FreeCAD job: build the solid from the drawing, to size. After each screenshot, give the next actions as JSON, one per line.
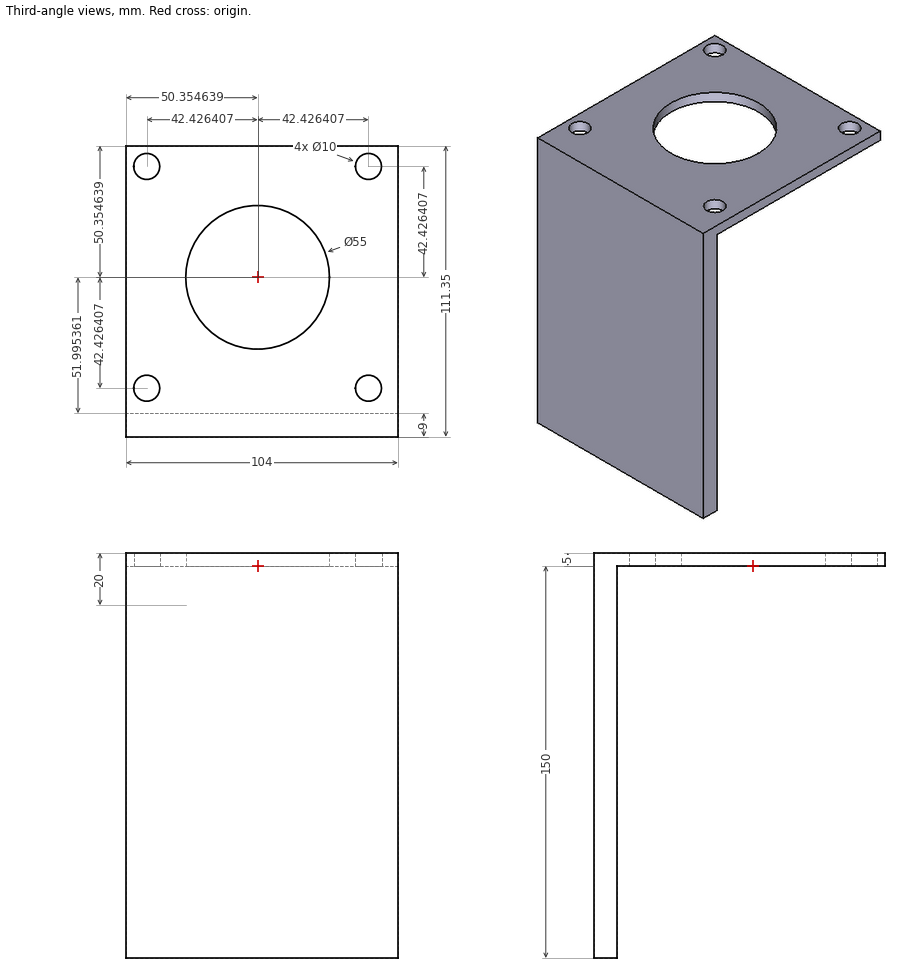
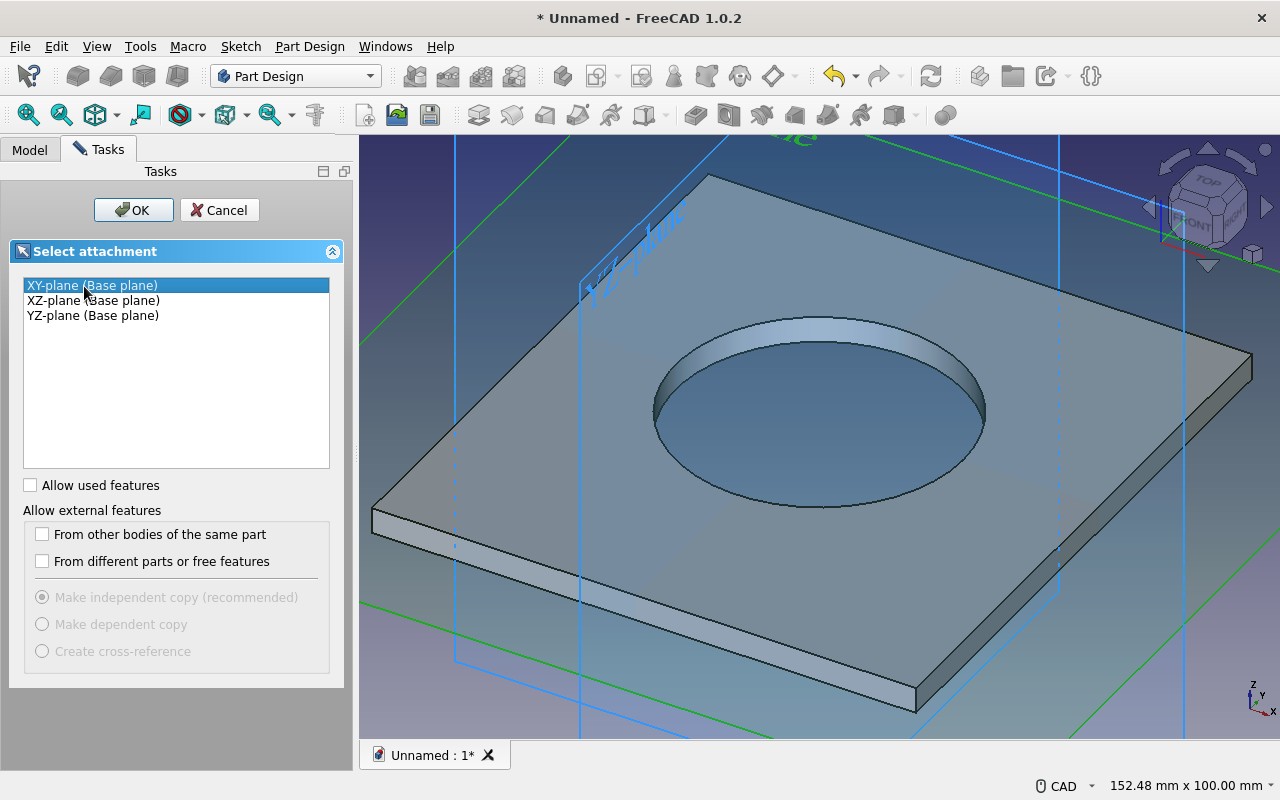
{"action": "left_click", "coordinate": [134, 210]}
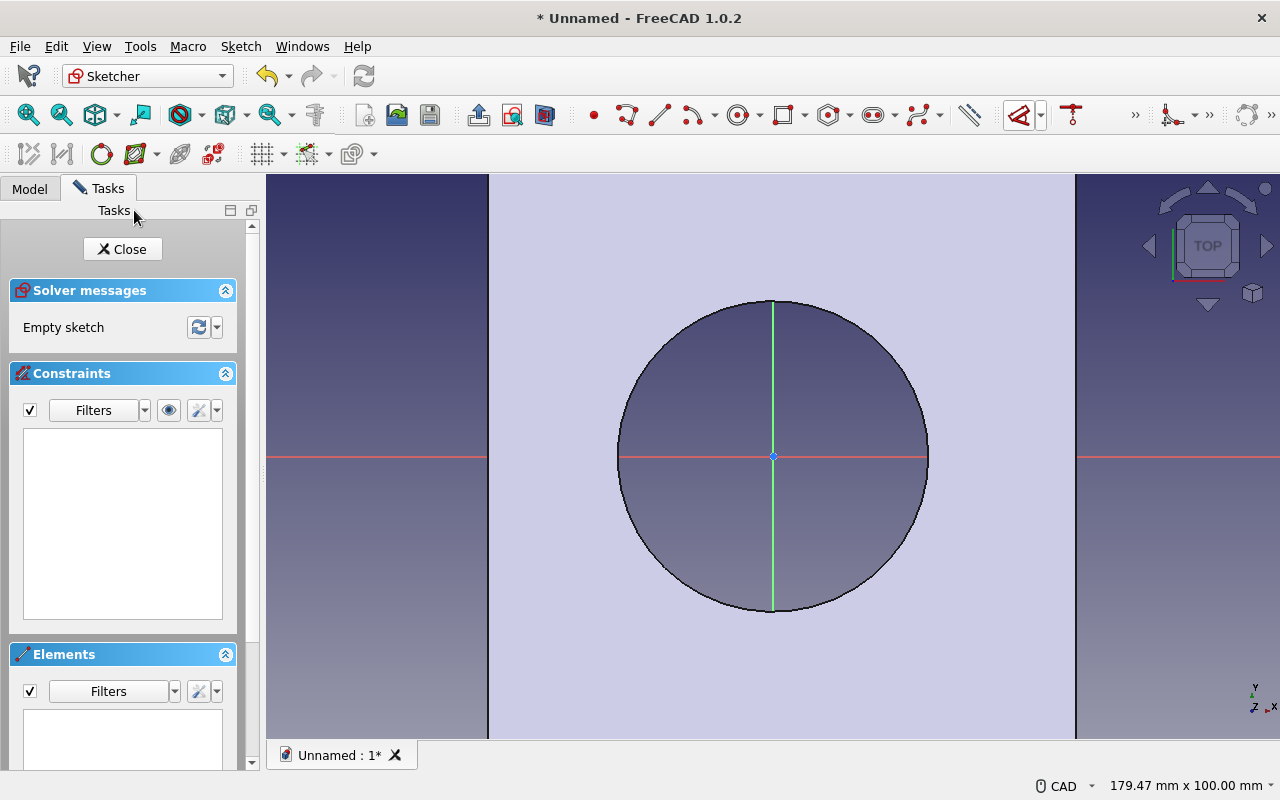
{"action": "left_click", "coordinate": [545, 116]}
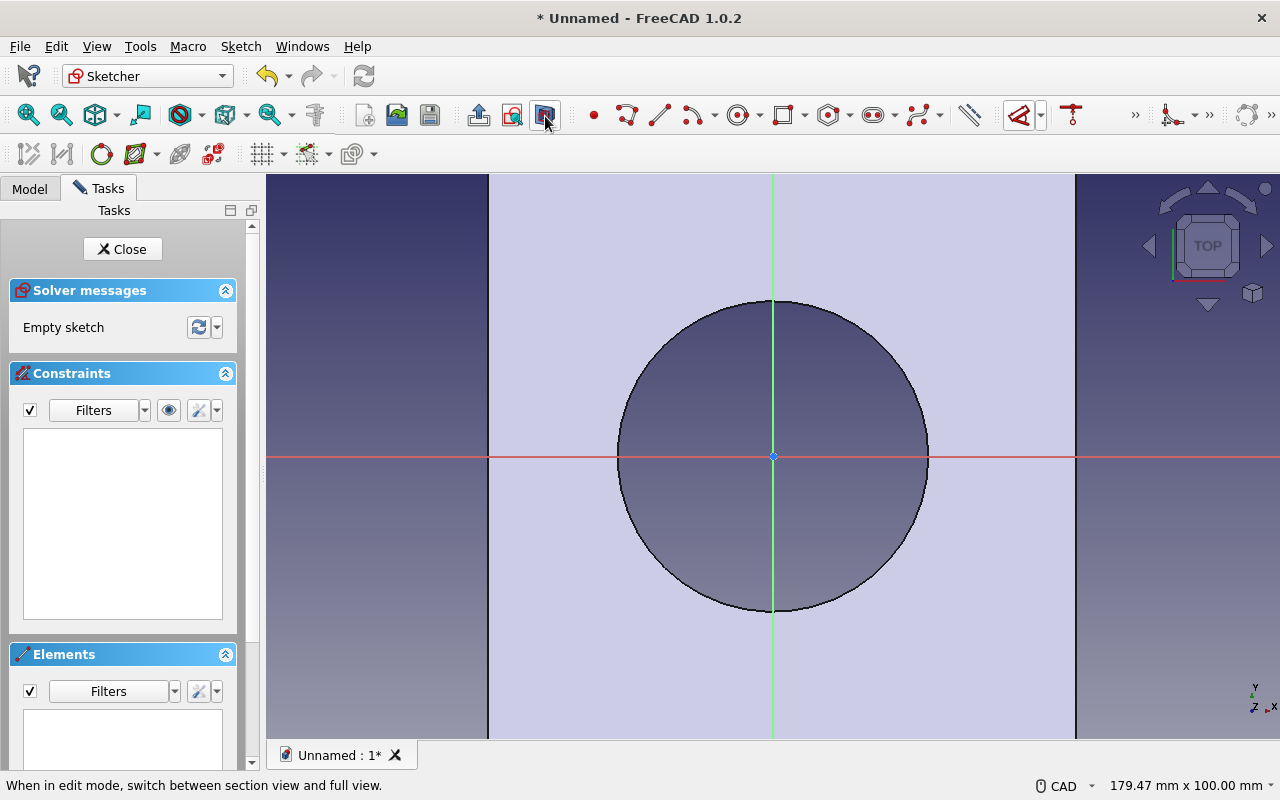
{"action": "scroll", "coordinate": [546, 202], "scroll_direction": "down", "scroll_amount": 2}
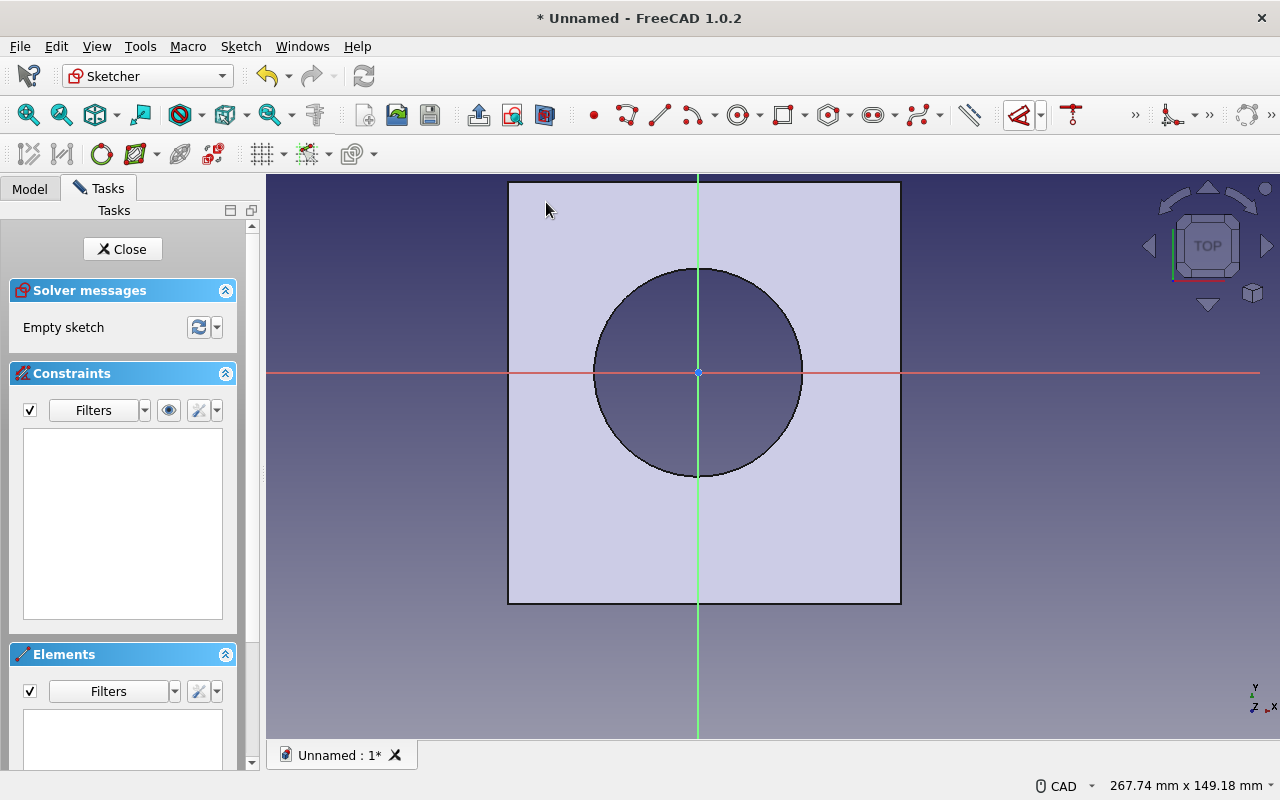
{"action": "scroll", "coordinate": [704, 552], "scroll_direction": "up", "scroll_amount": 2}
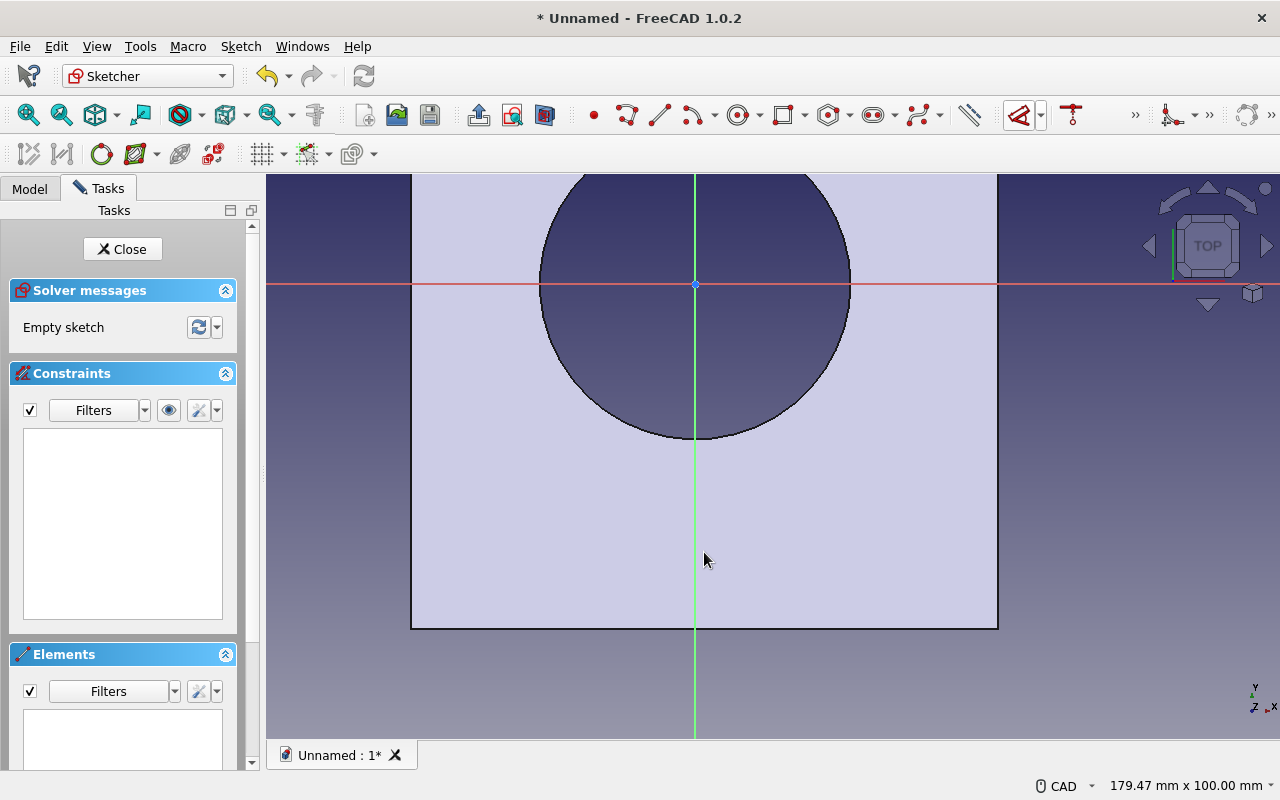
{"action": "left_click", "coordinate": [782, 116]}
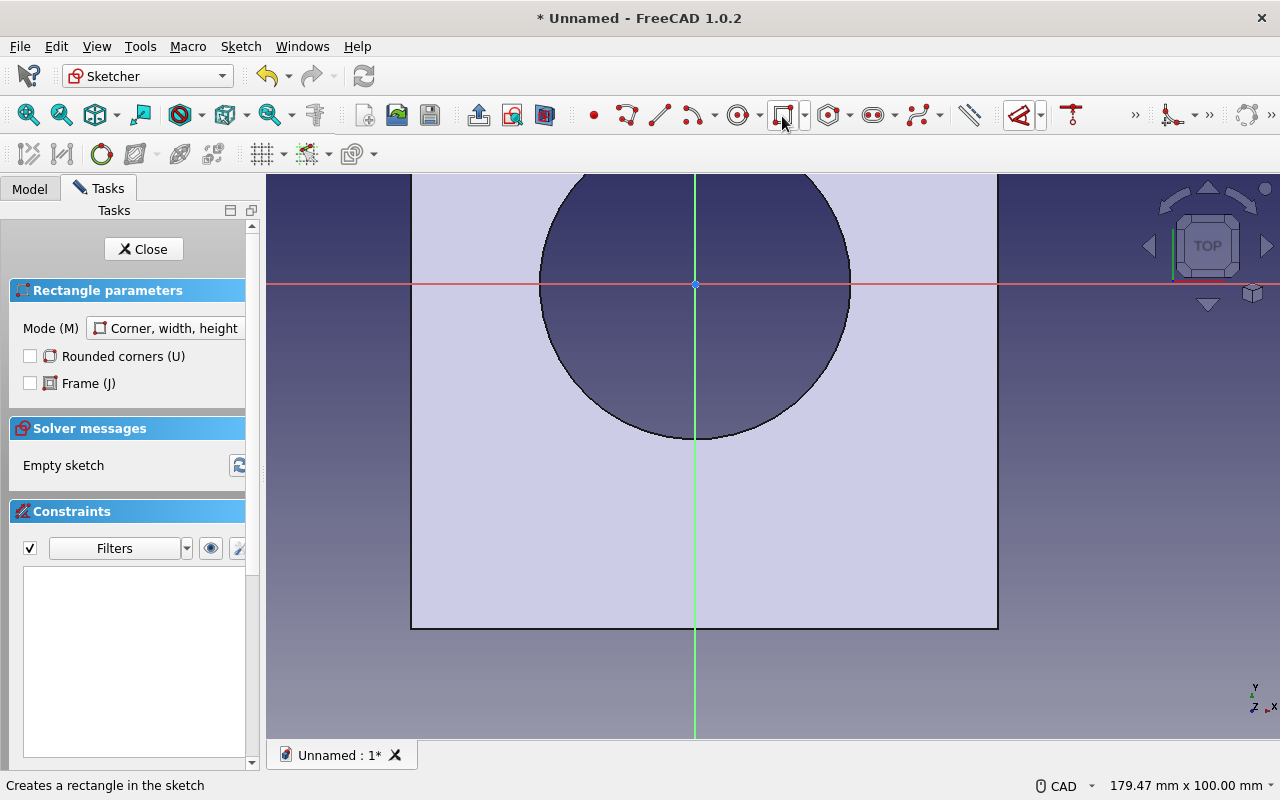
{"action": "left_click", "coordinate": [411, 578]}
{"action": "mouse_move", "coordinate": [998, 629]}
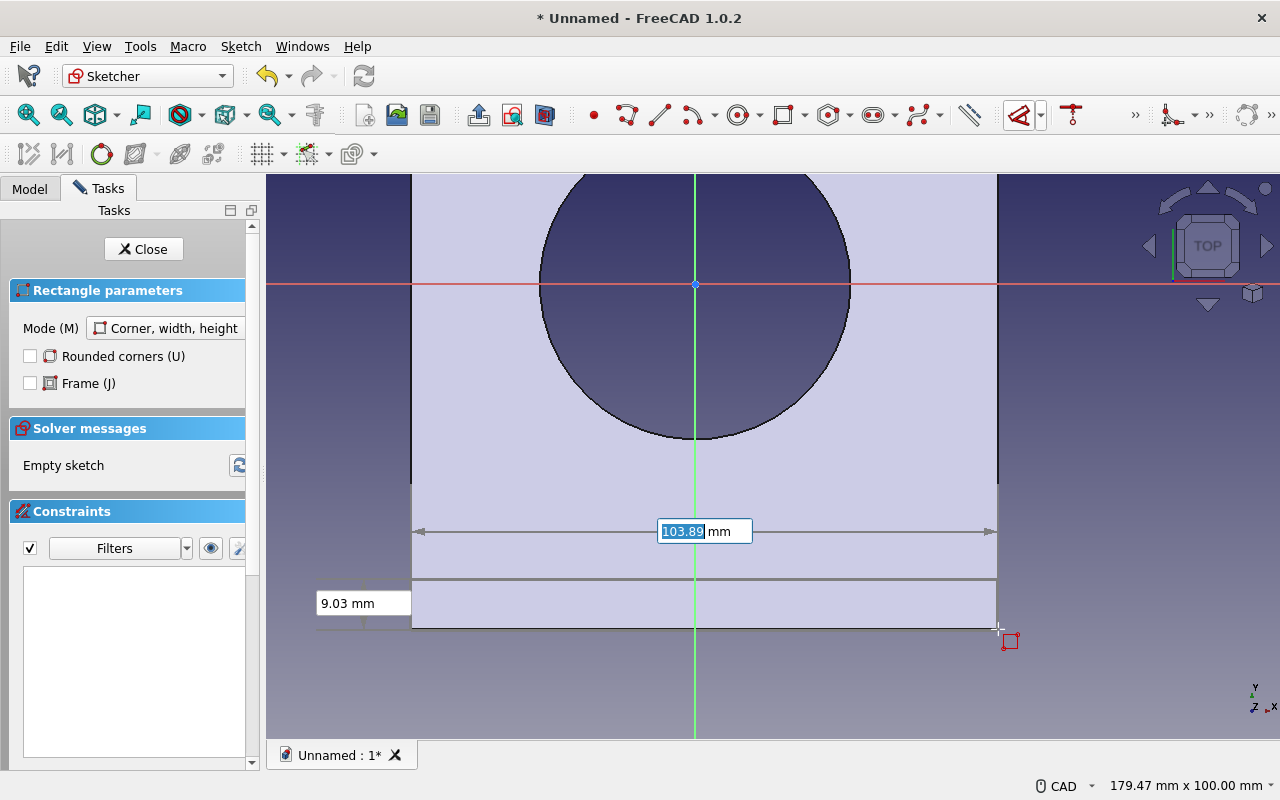
{"action": "type", "text": "104"}
{"action": "key", "text": "Tab"}
{"action": "type", "text": "9"}
{"action": "key", "text": "Return"}
{"action": "key", "text": "Escape"}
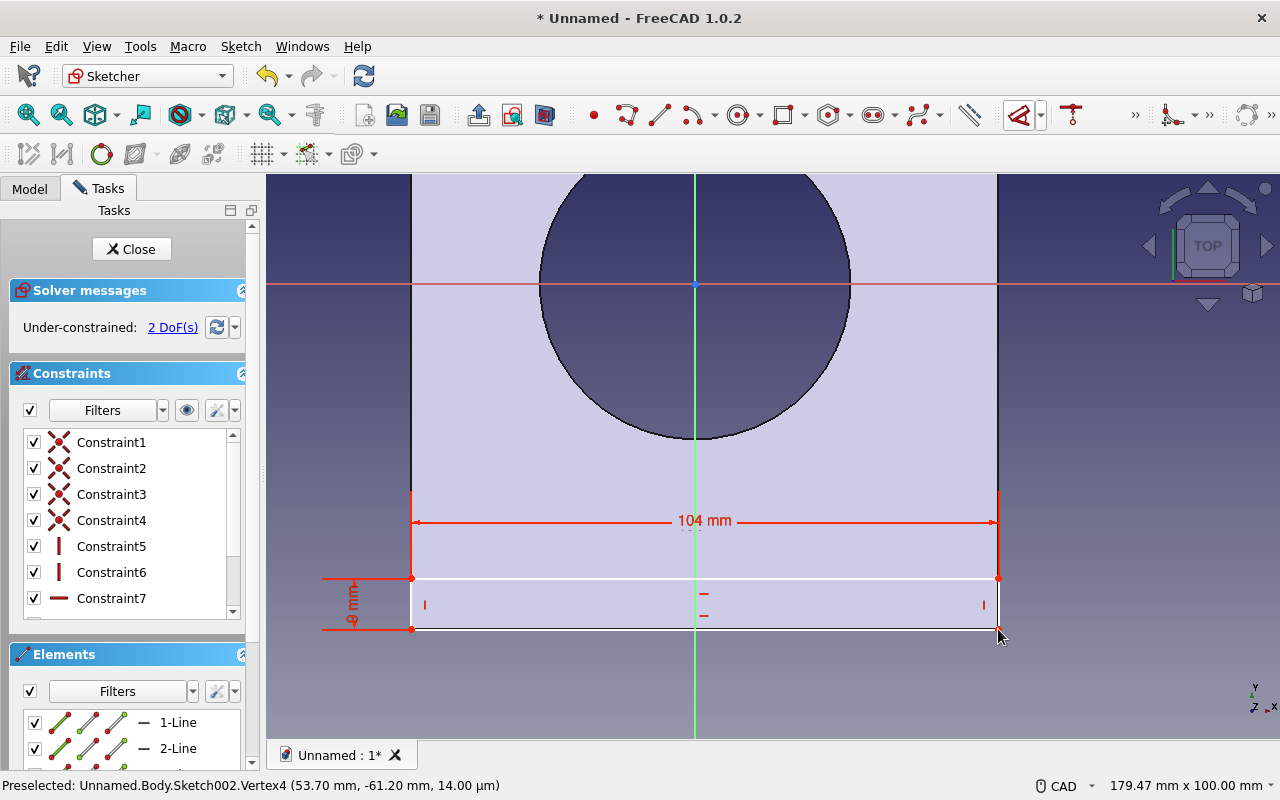
{"action": "left_click", "coordinate": [411, 579]}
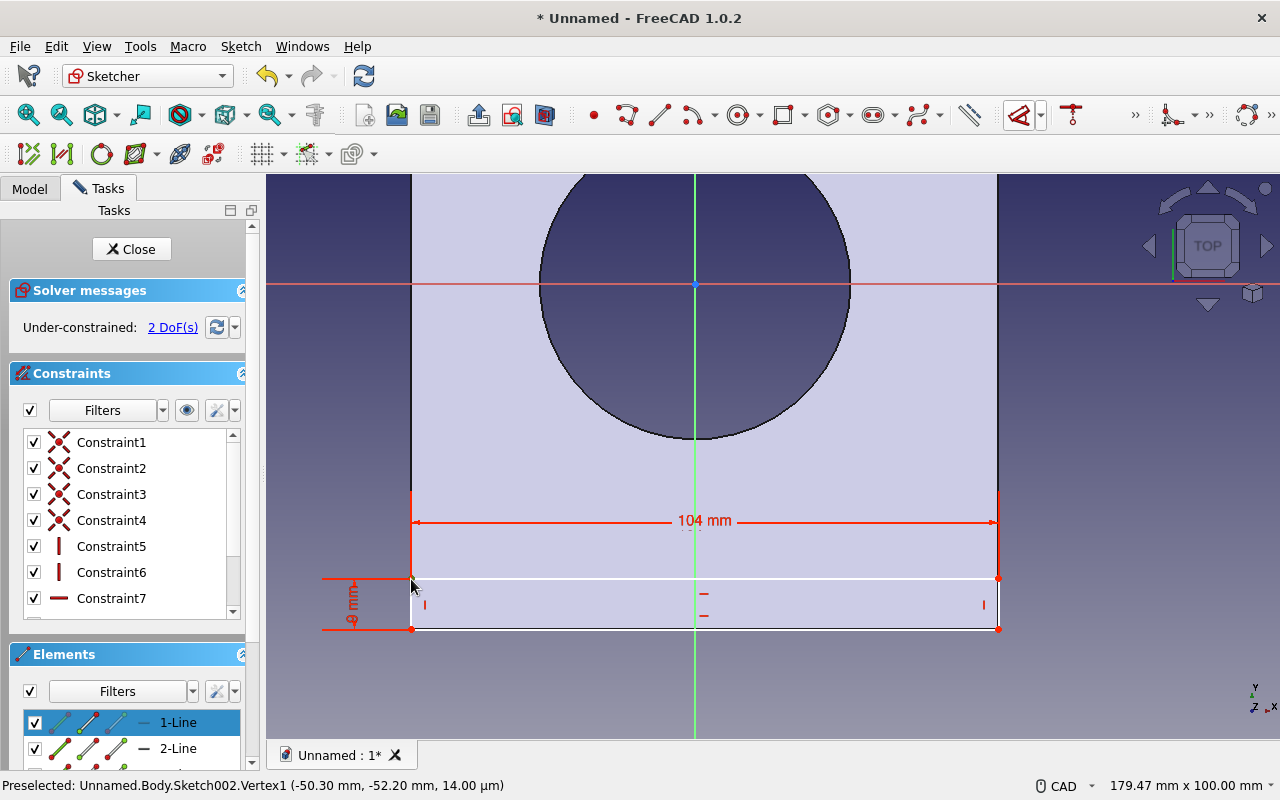
{"action": "key", "text": "l"}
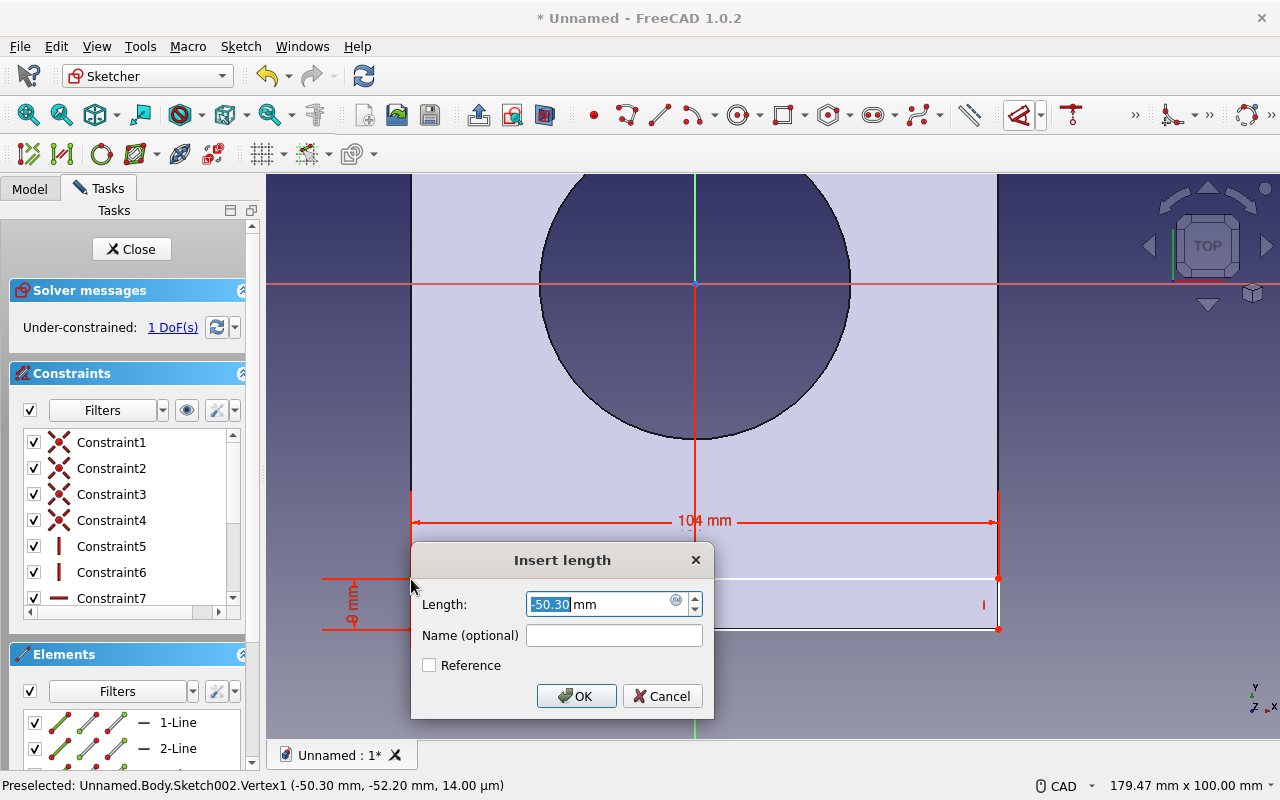
{"action": "type", "text": "-50.354639"}
{"action": "key", "text": "Return"}